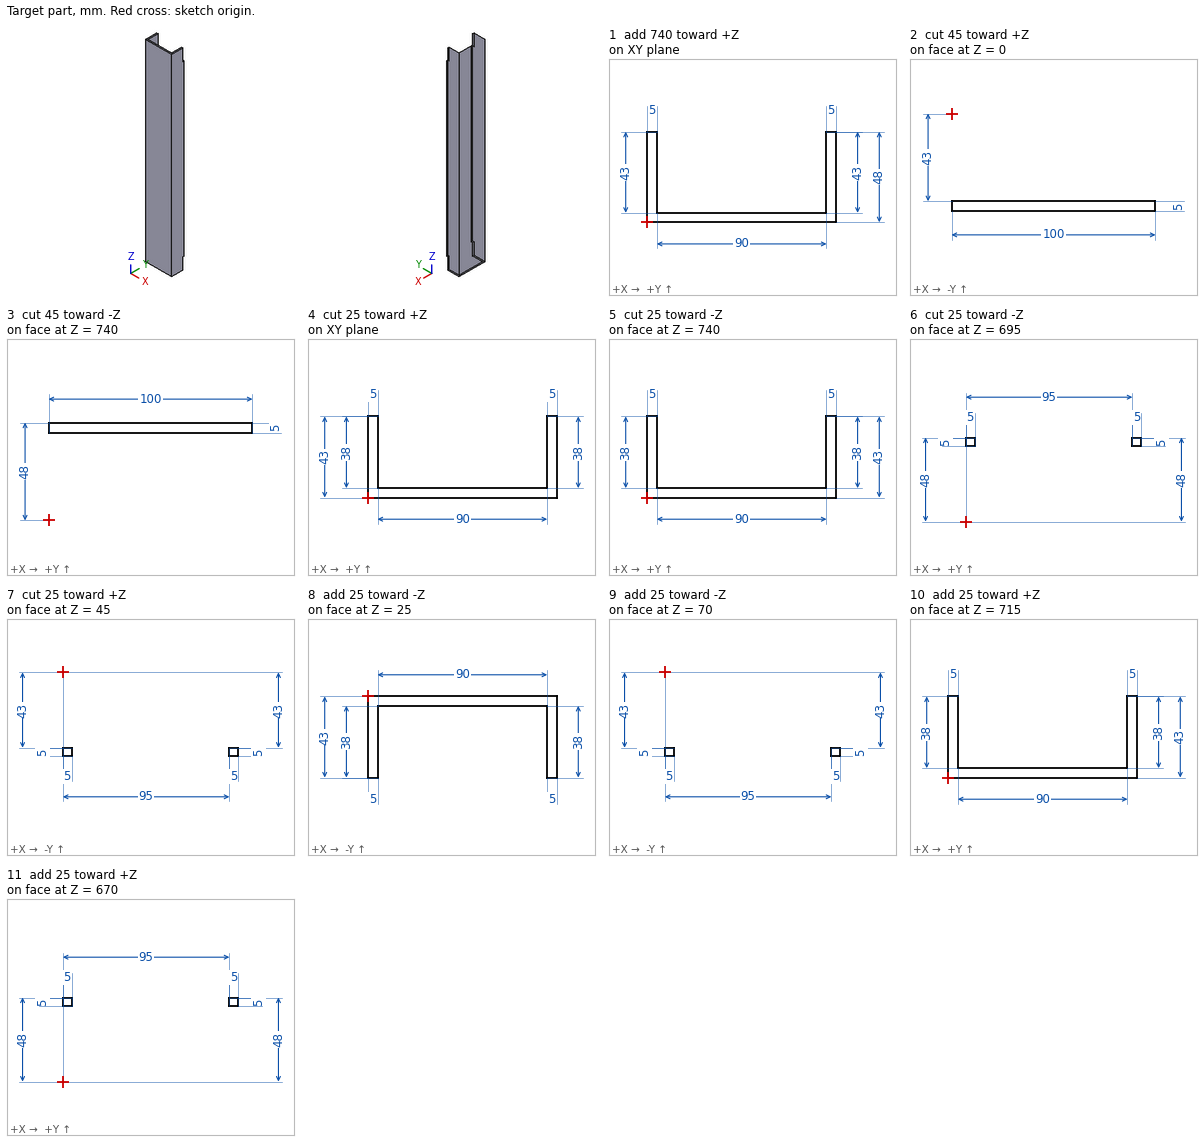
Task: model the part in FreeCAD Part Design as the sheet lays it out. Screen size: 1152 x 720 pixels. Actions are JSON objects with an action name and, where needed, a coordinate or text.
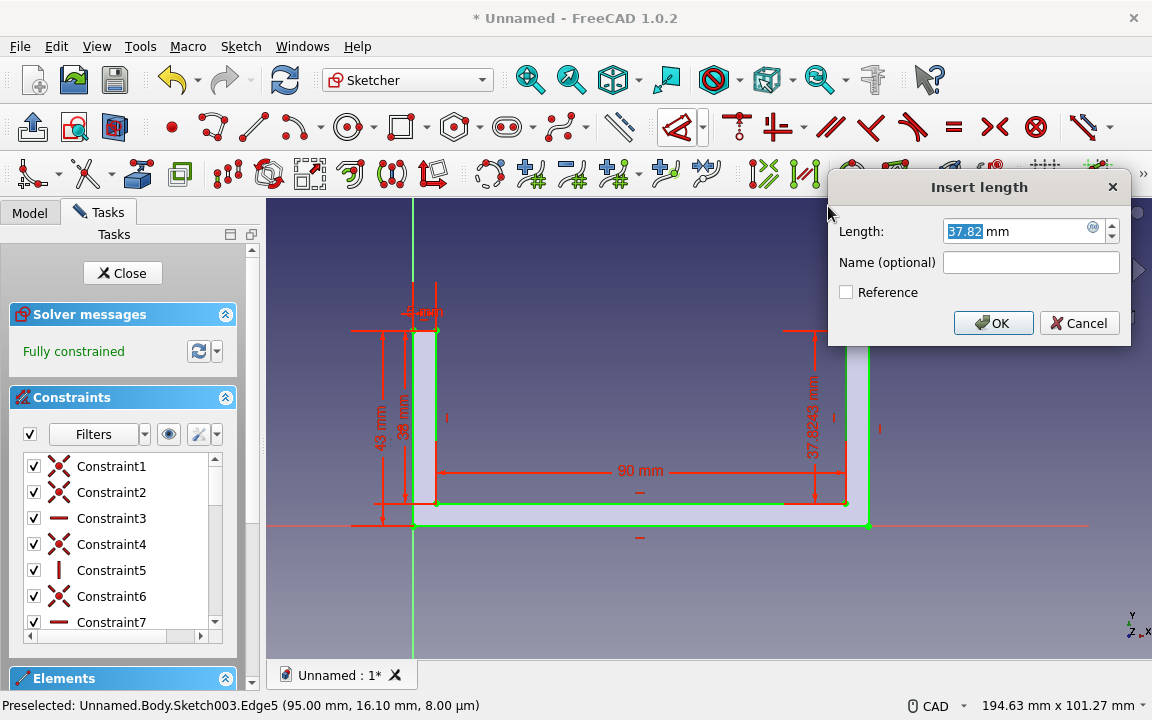
{"action": "type", "text": "38"}
{"action": "key", "text": "Return"}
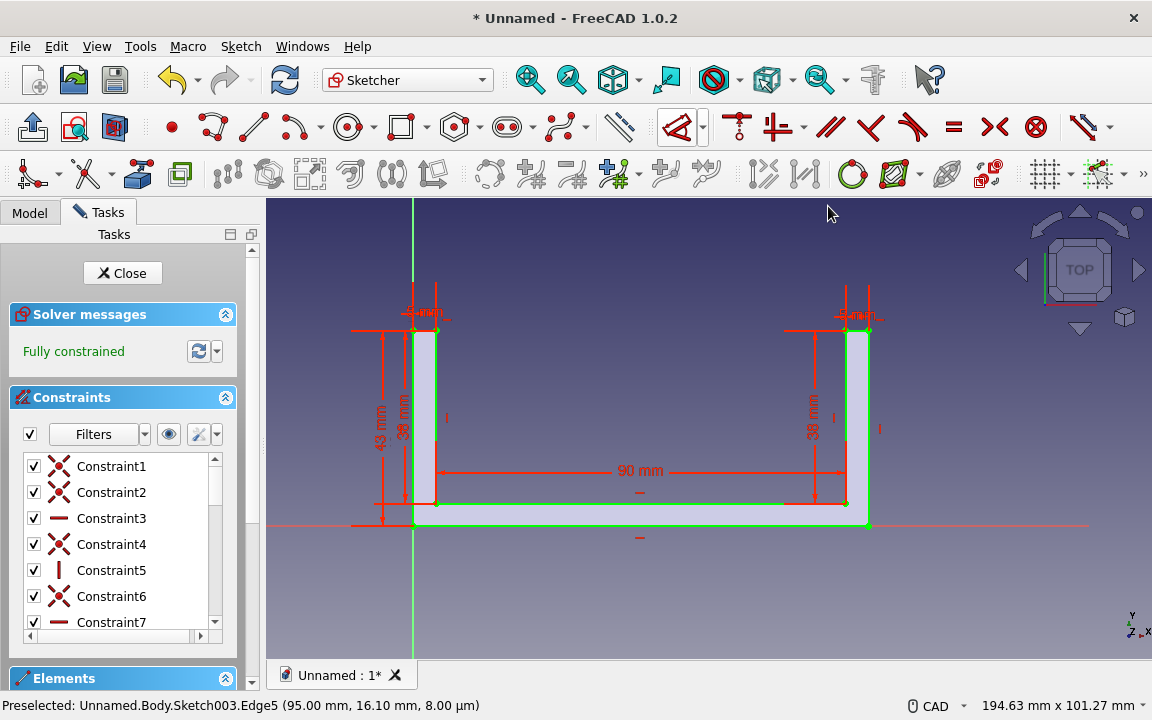
{"action": "left_click", "coordinate": [123, 273]}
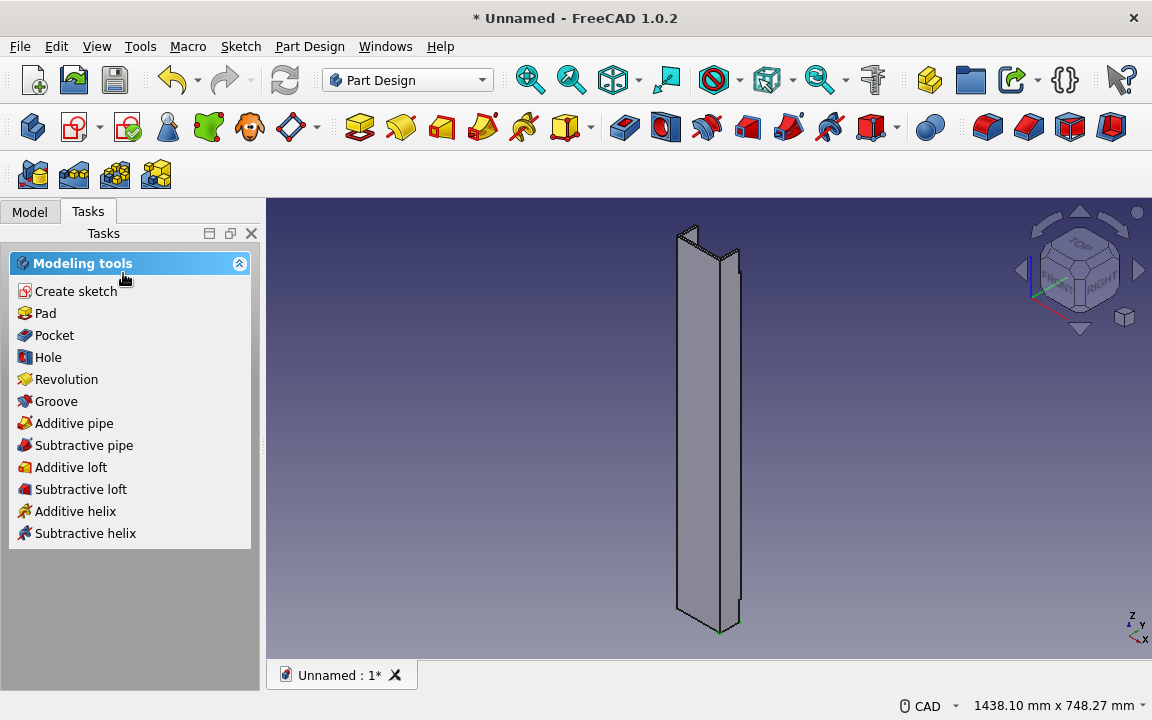
{"action": "left_click", "coordinate": [625, 128]}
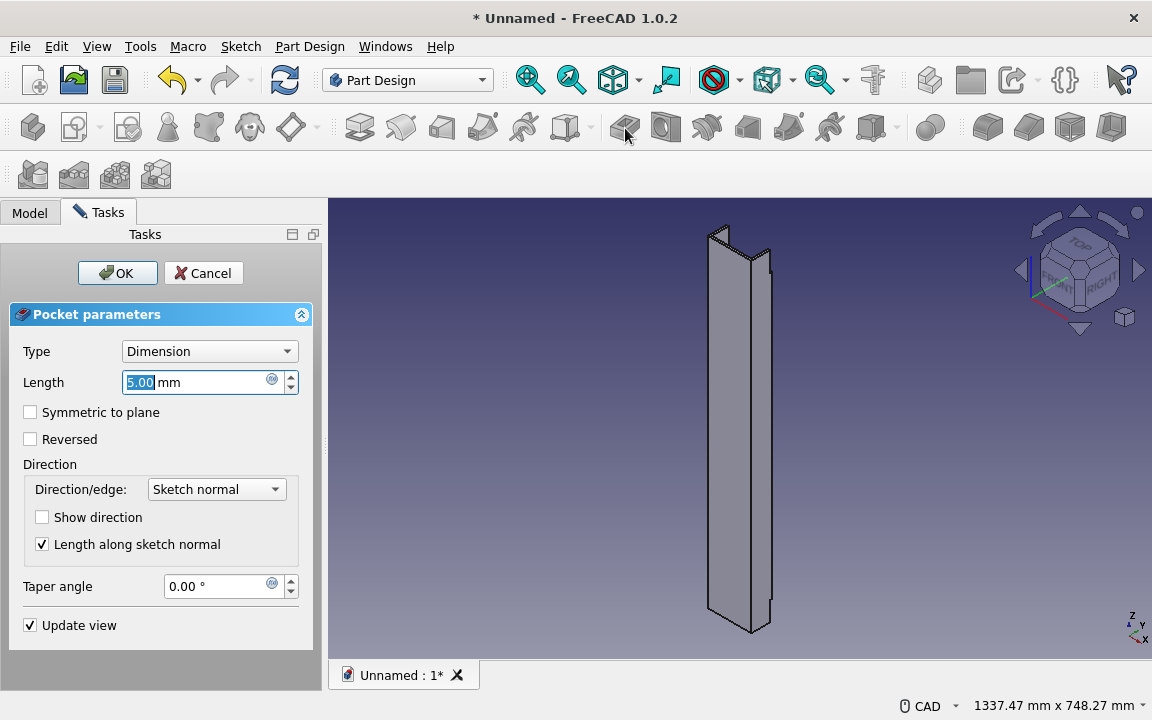
{"action": "type", "text": "25"}
{"action": "key", "text": "Tab"}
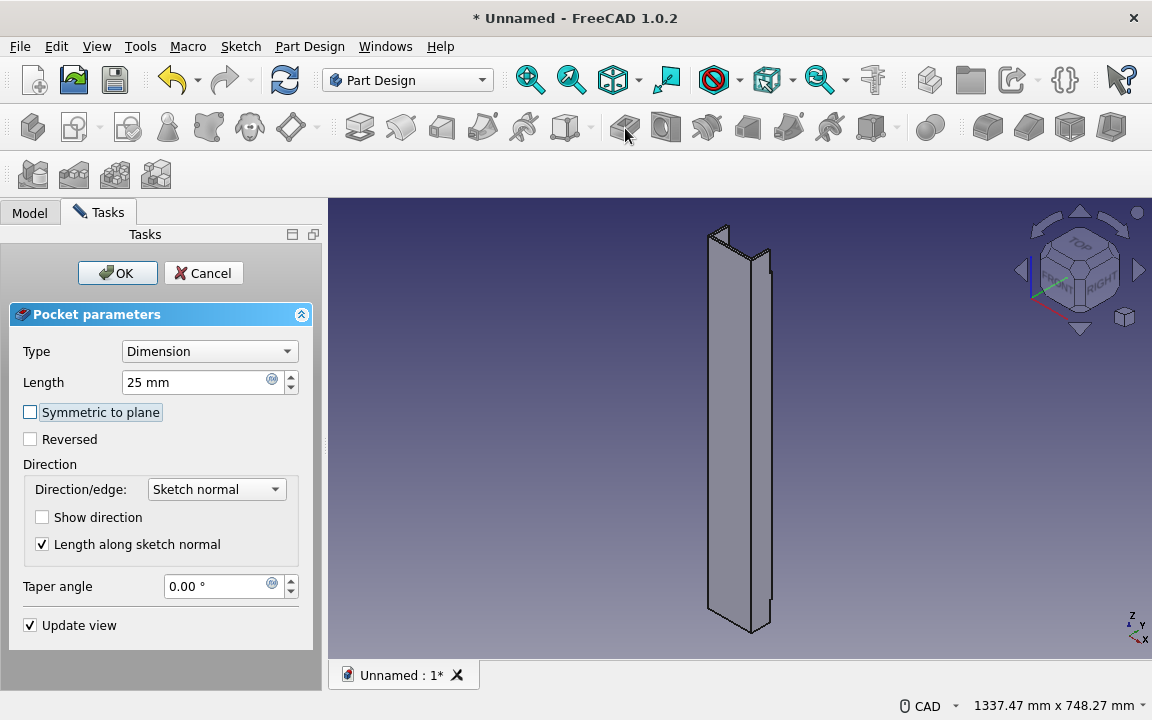
{"action": "left_click", "coordinate": [31, 439]}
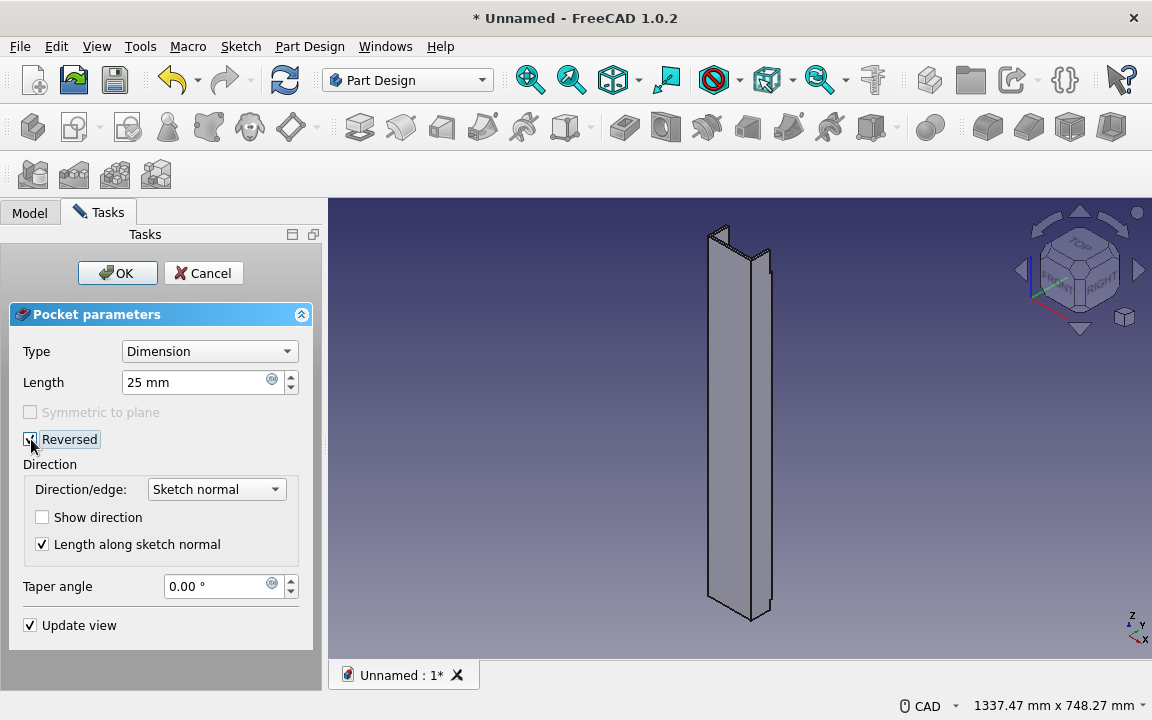
{"action": "left_click", "coordinate": [118, 273]}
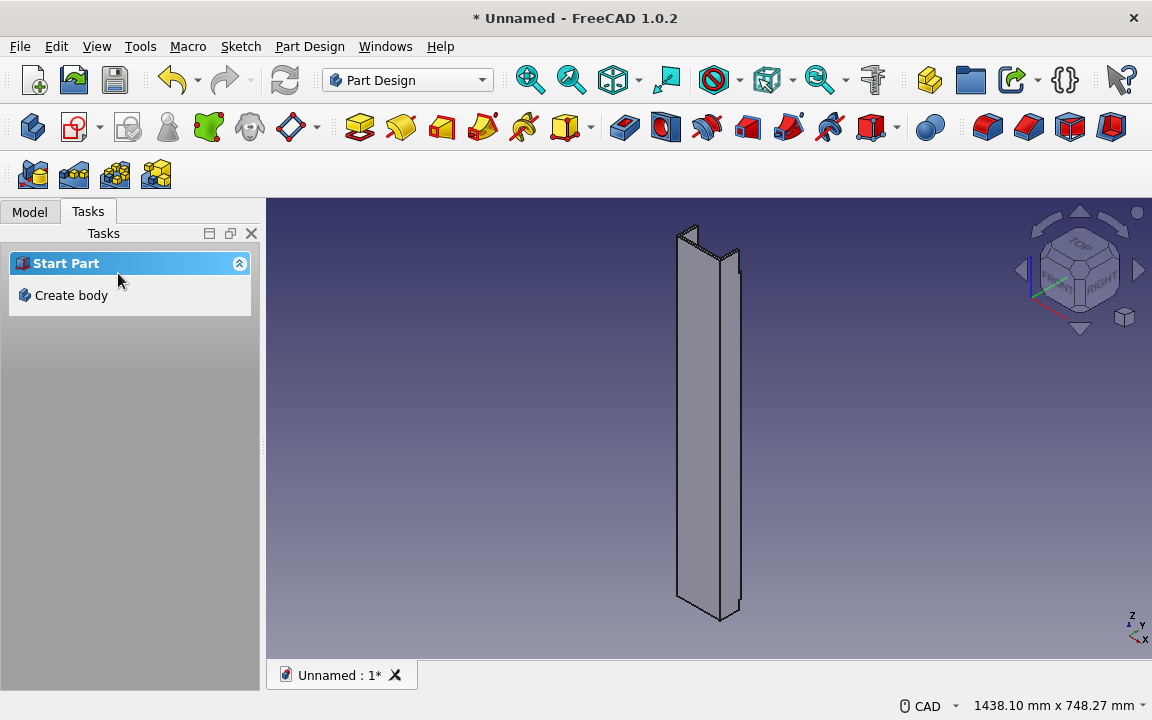
{"action": "scroll", "coordinate": [719, 257], "scroll_direction": "up", "scroll_amount": 12}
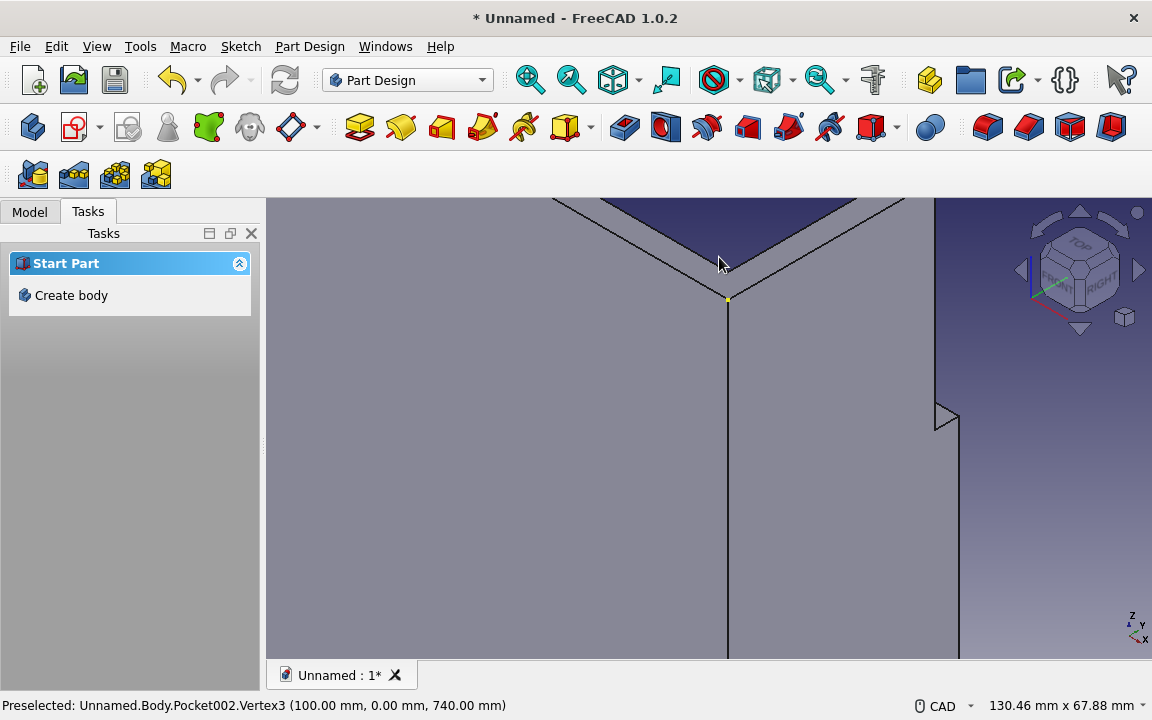
{"action": "left_click", "coordinate": [709, 270]}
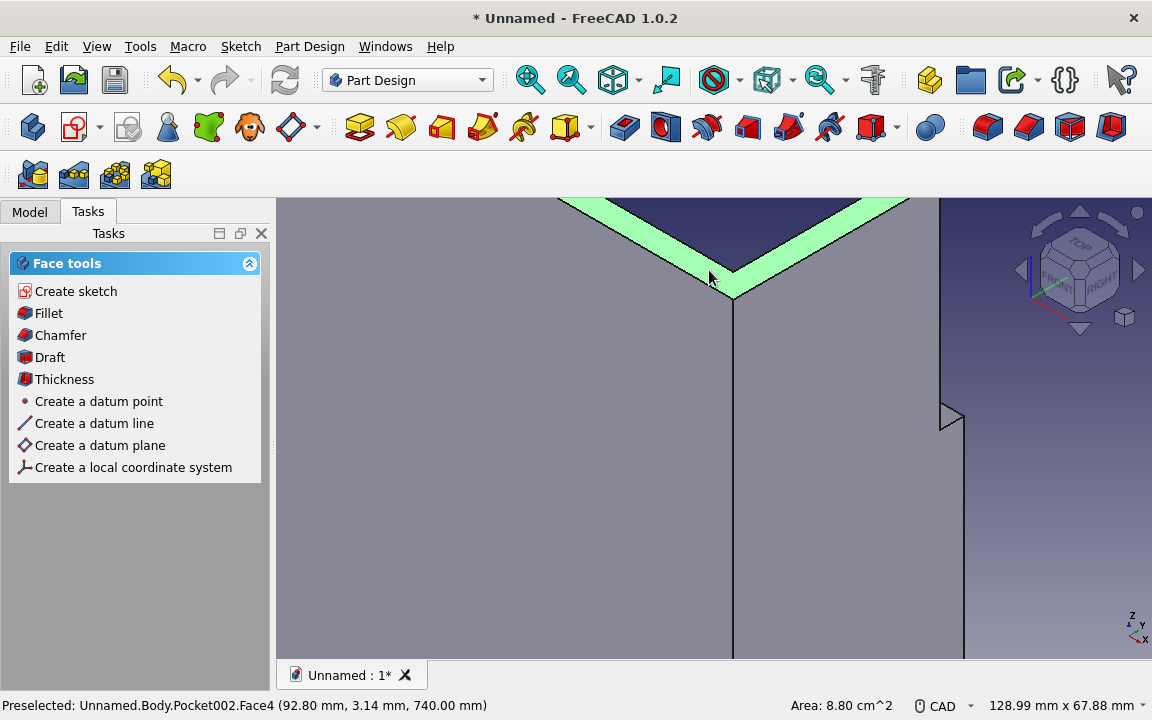
{"action": "left_click", "coordinate": [74, 128]}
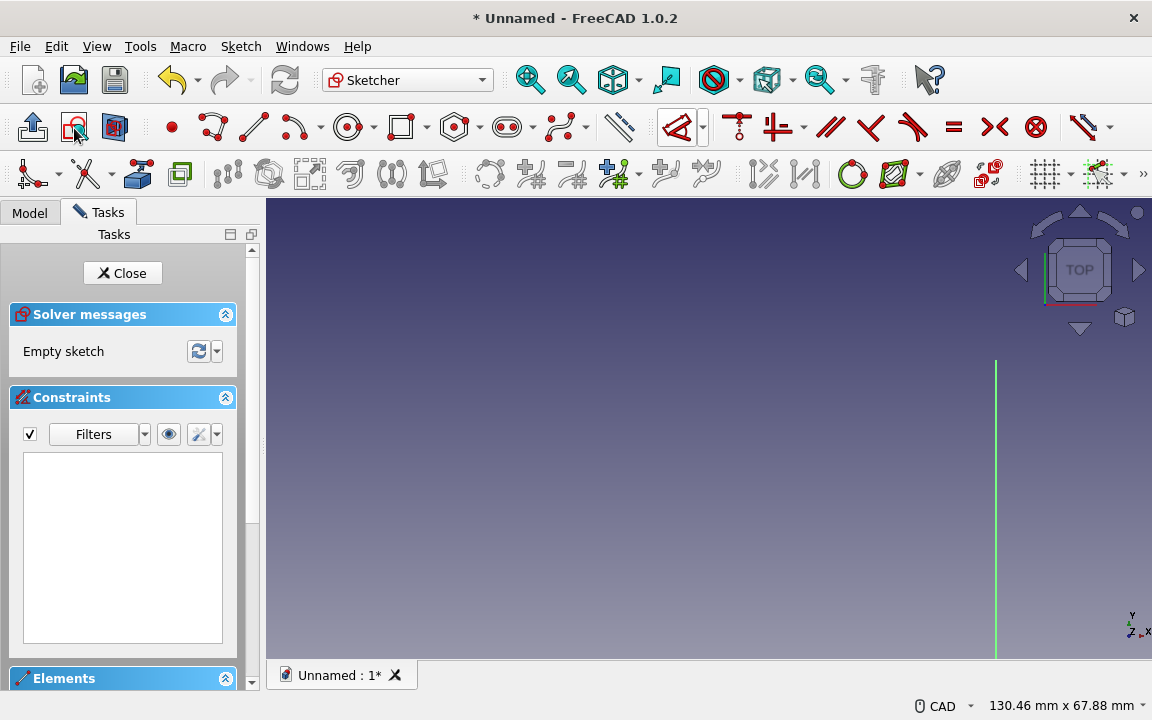
{"action": "scroll", "coordinate": [640, 428], "scroll_direction": "down", "scroll_amount": 5}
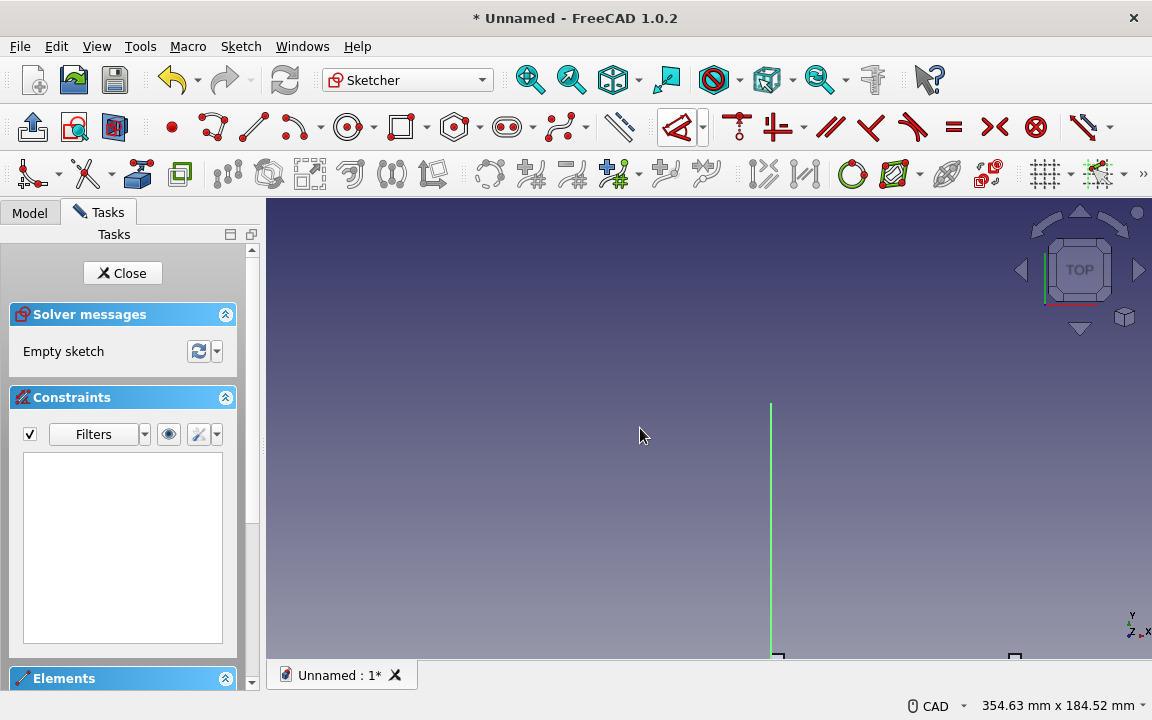
{"action": "scroll", "coordinate": [640, 428], "scroll_direction": "down", "scroll_amount": 5}